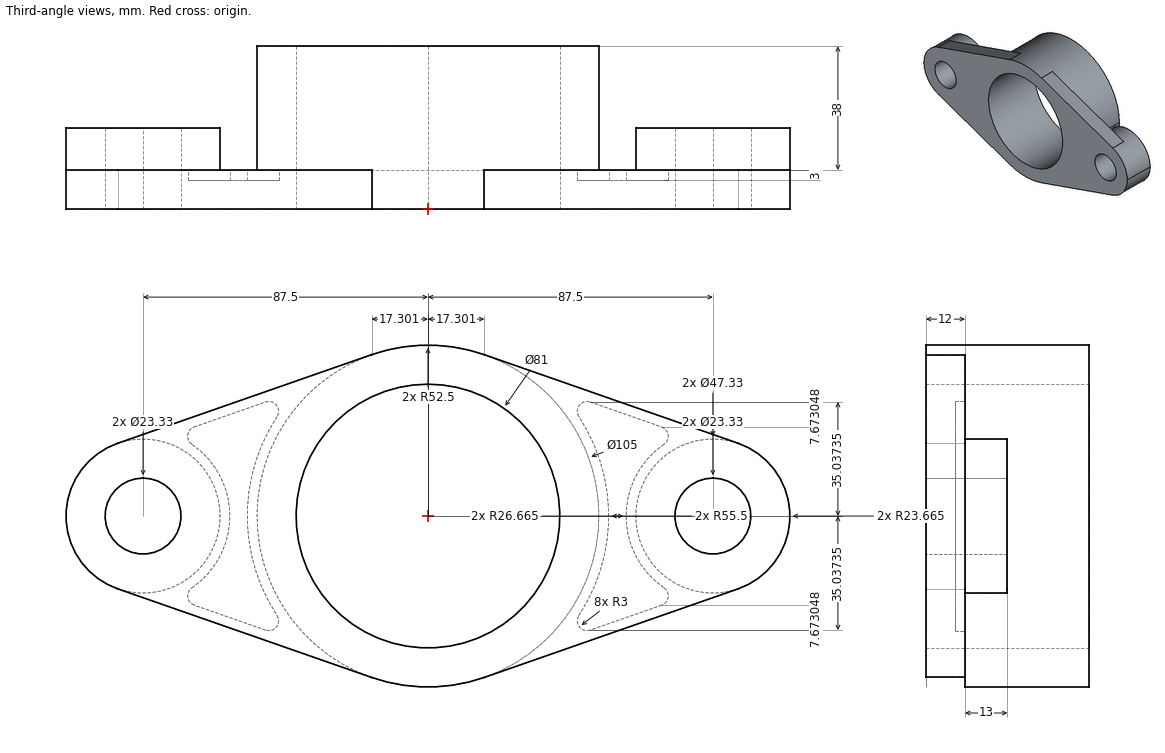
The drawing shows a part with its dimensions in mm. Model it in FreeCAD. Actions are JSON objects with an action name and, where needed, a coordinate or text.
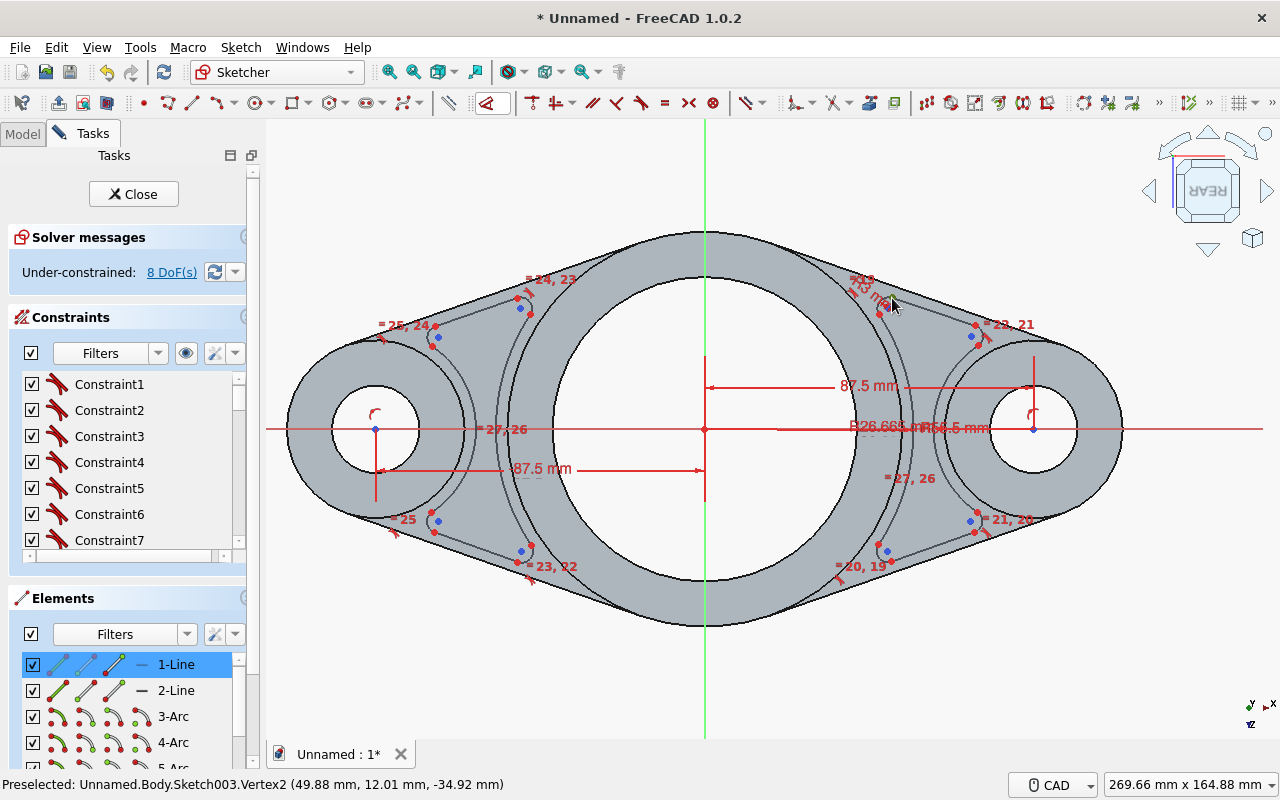
{"action": "left_click", "coordinate": [504, 104]}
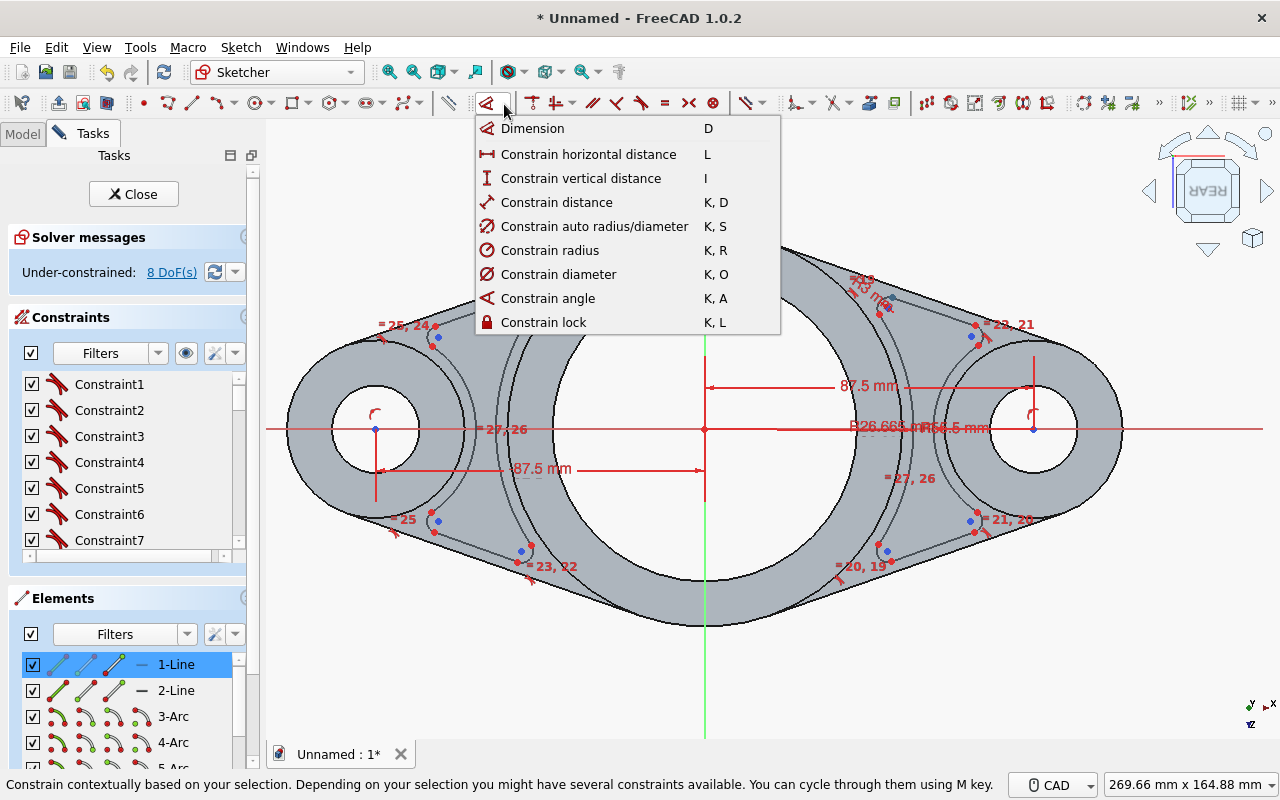
{"action": "left_click", "coordinate": [628, 178]}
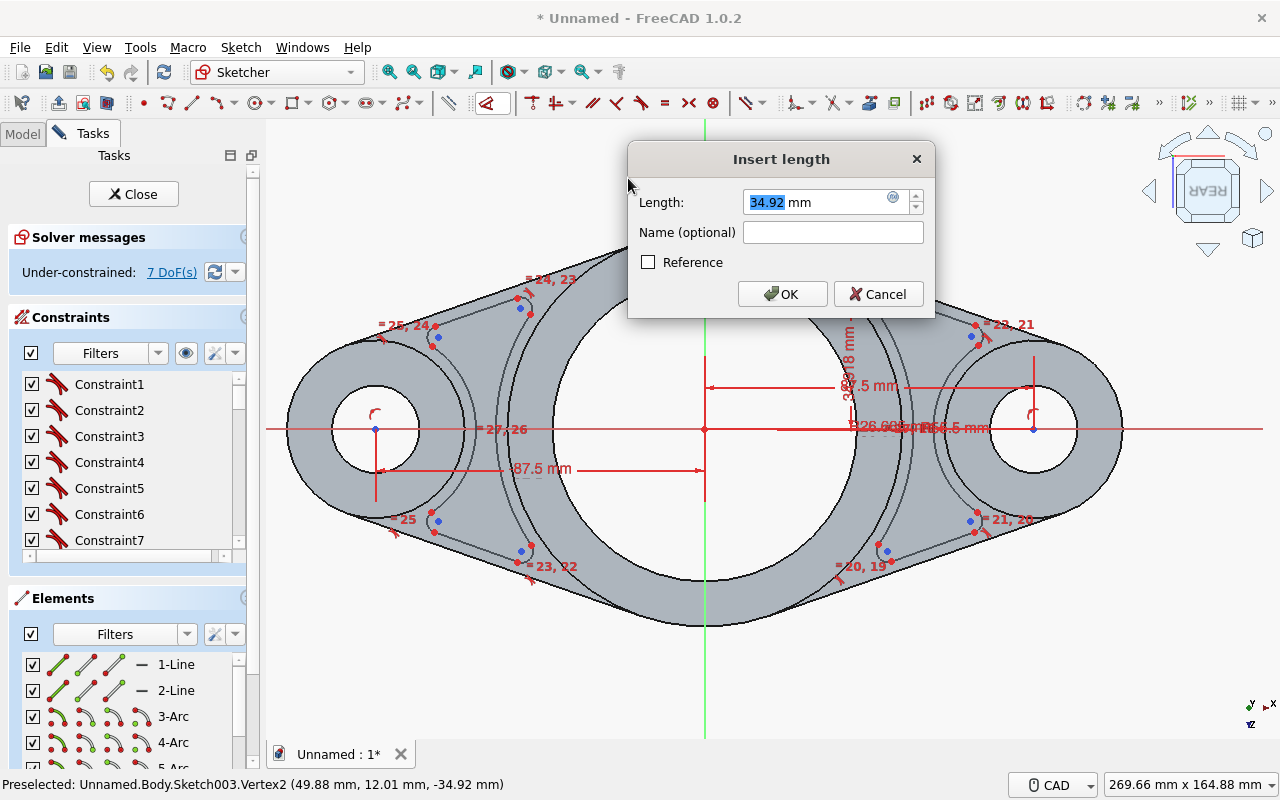
{"action": "type", "text": "35.03735"}
{"action": "key", "text": "Return"}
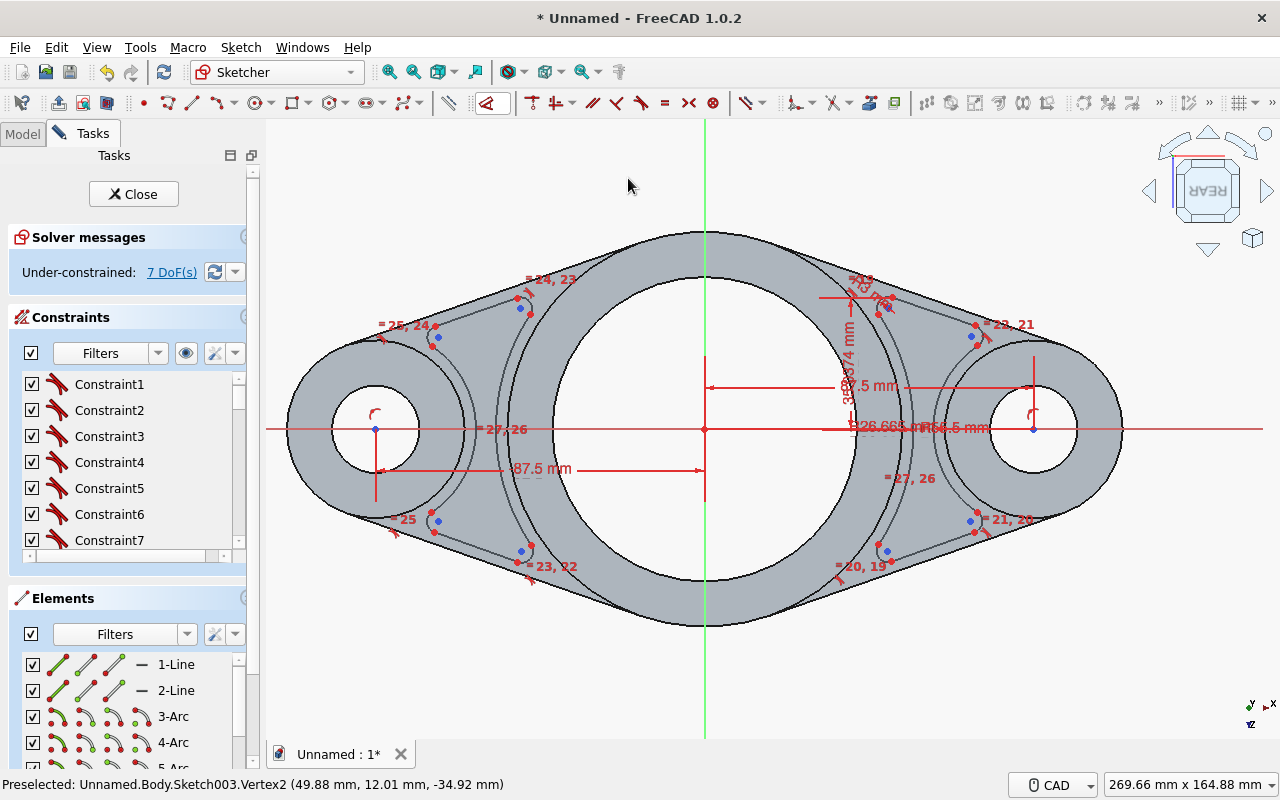
{"action": "left_click", "coordinate": [892, 562]}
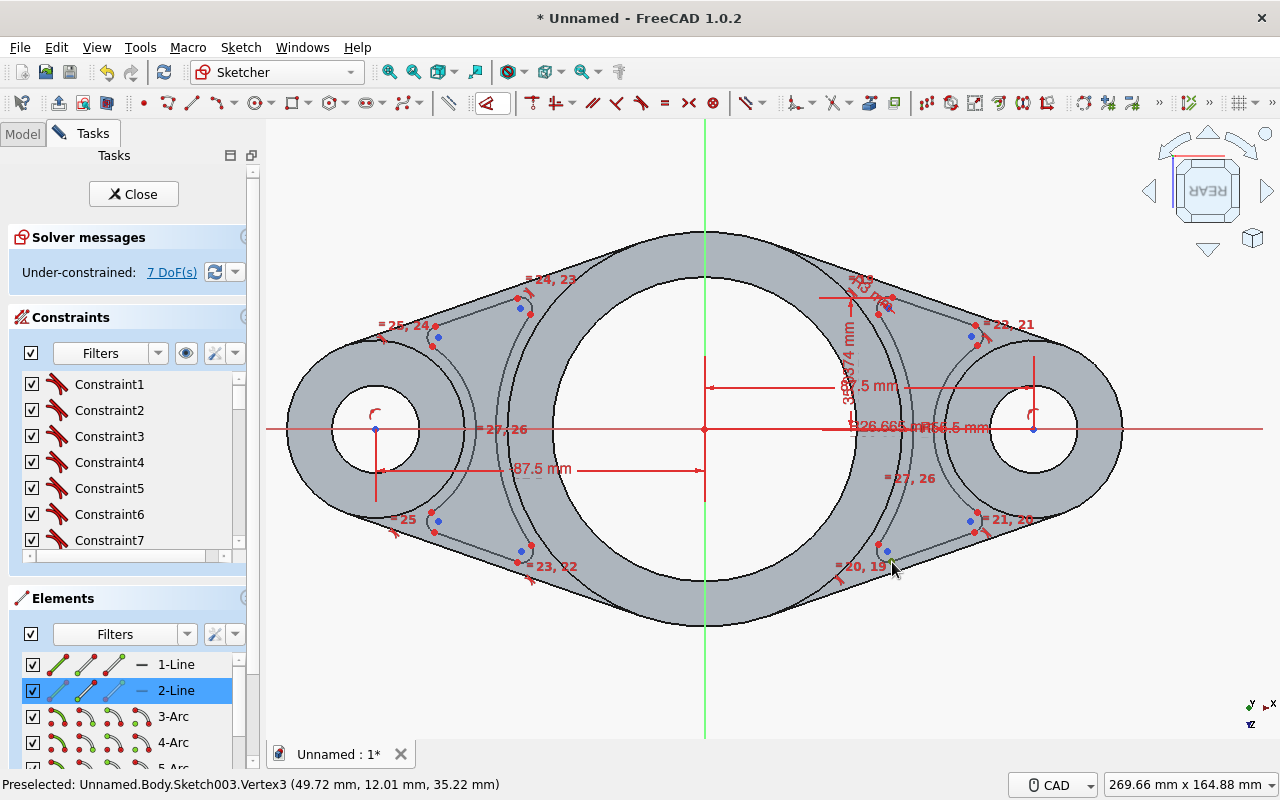
{"action": "left_click", "coordinate": [504, 104]}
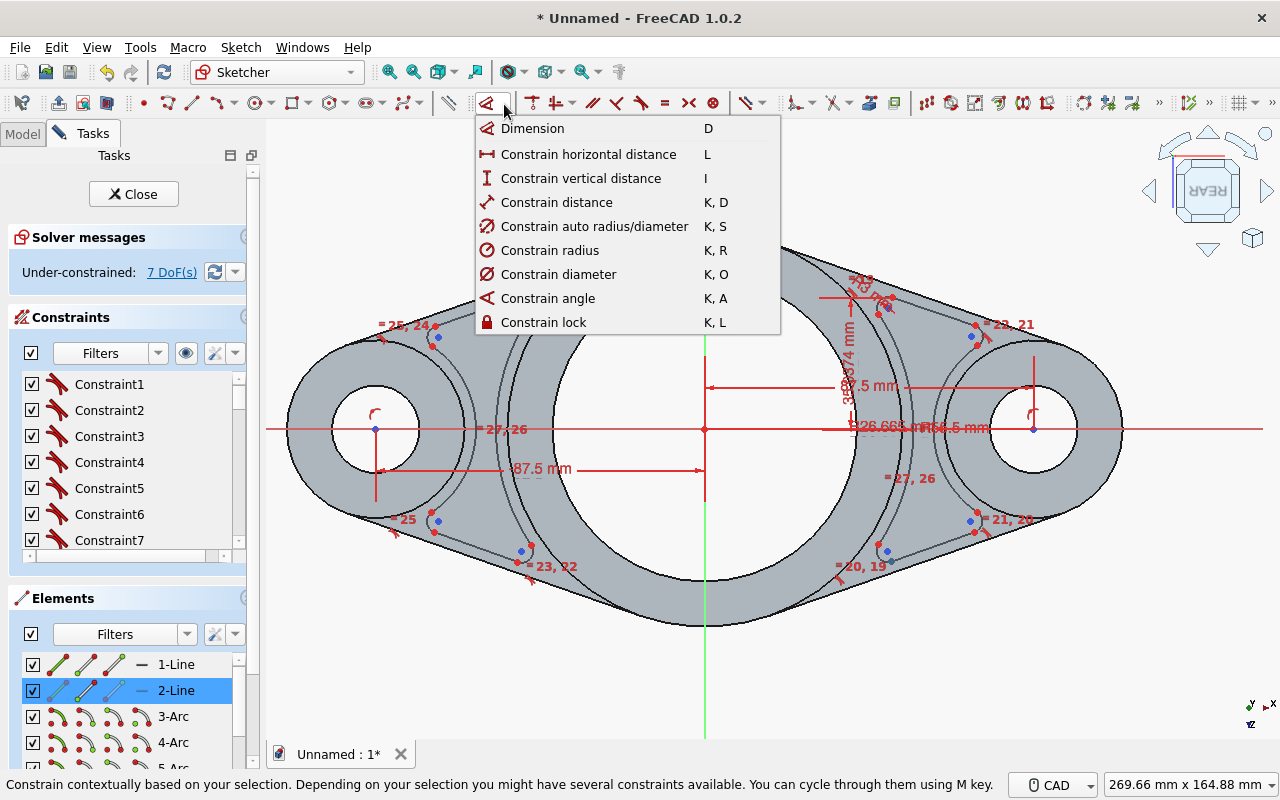
{"action": "left_click", "coordinate": [628, 178]}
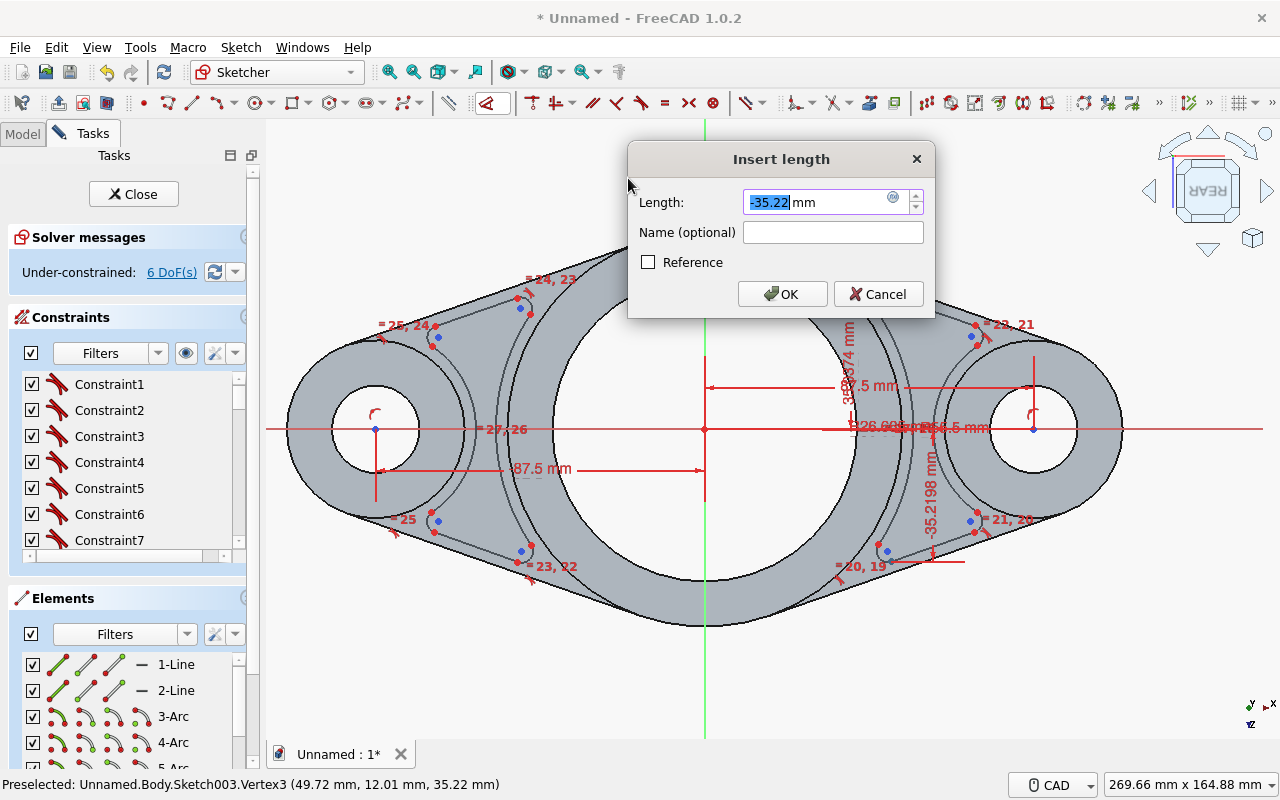
{"action": "type", "text": "-35.03735"}
{"action": "key", "text": "Return"}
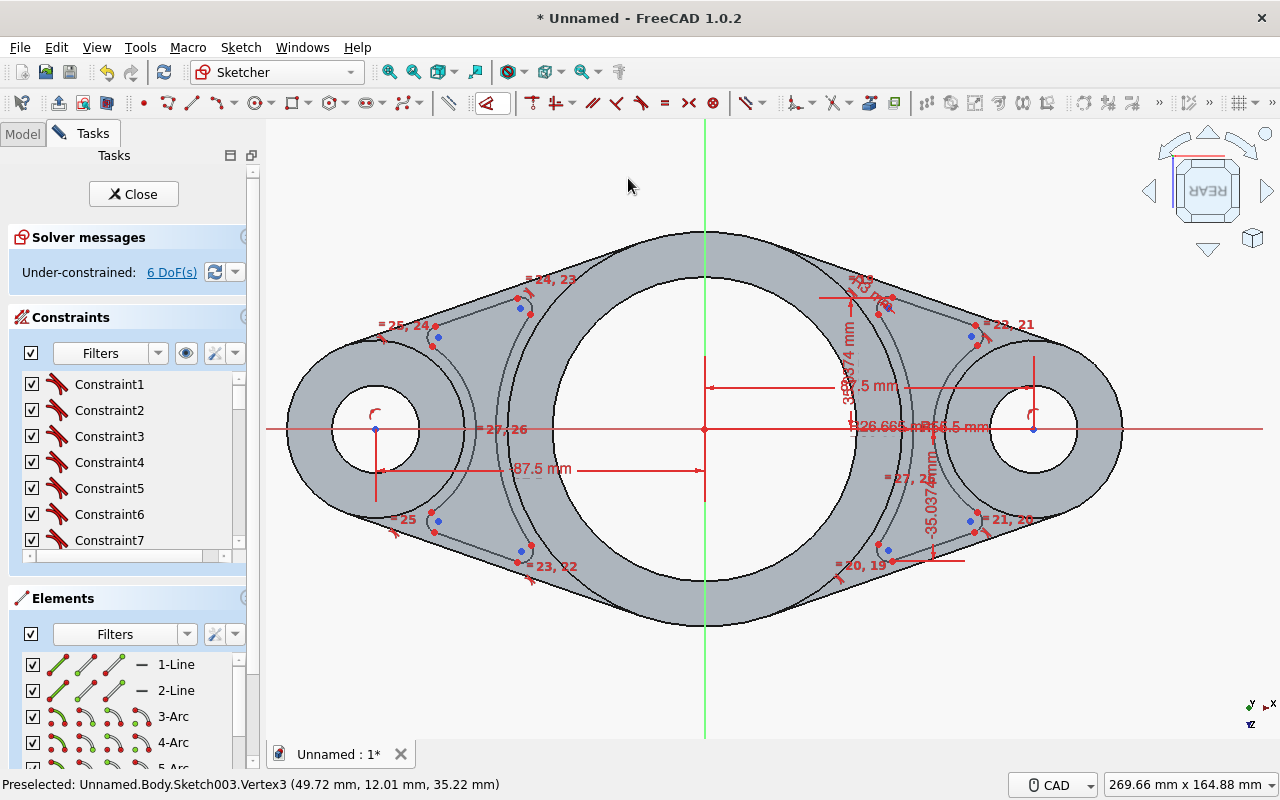
{"action": "left_click", "coordinate": [518, 562]}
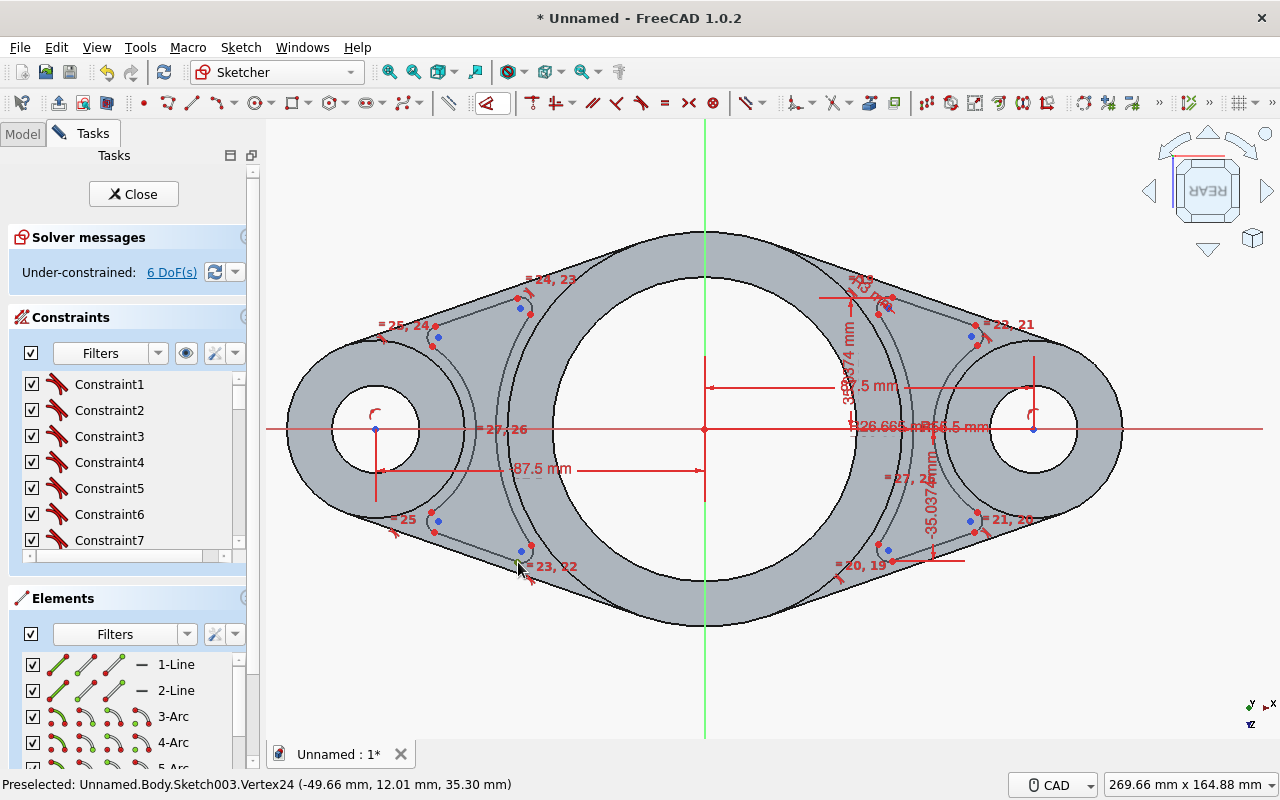
{"action": "left_click", "coordinate": [504, 104]}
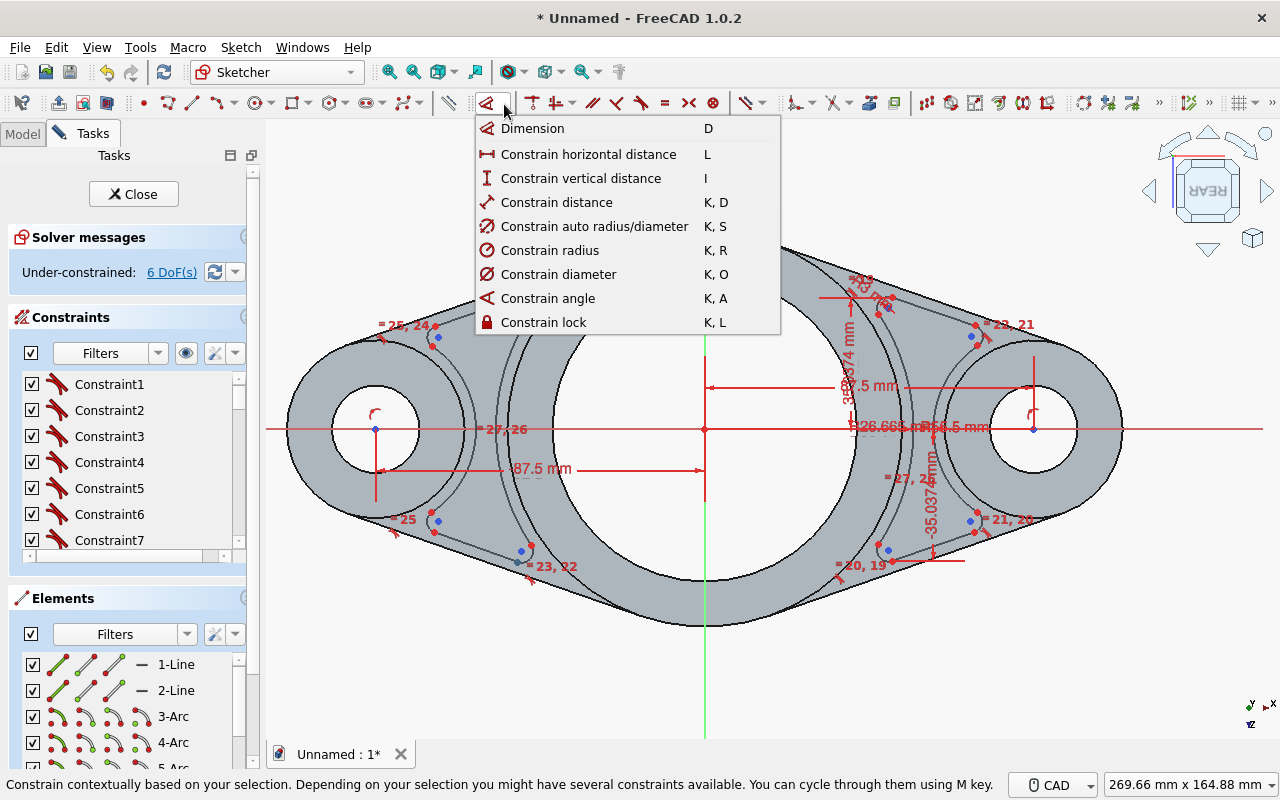
{"action": "left_click", "coordinate": [628, 178]}